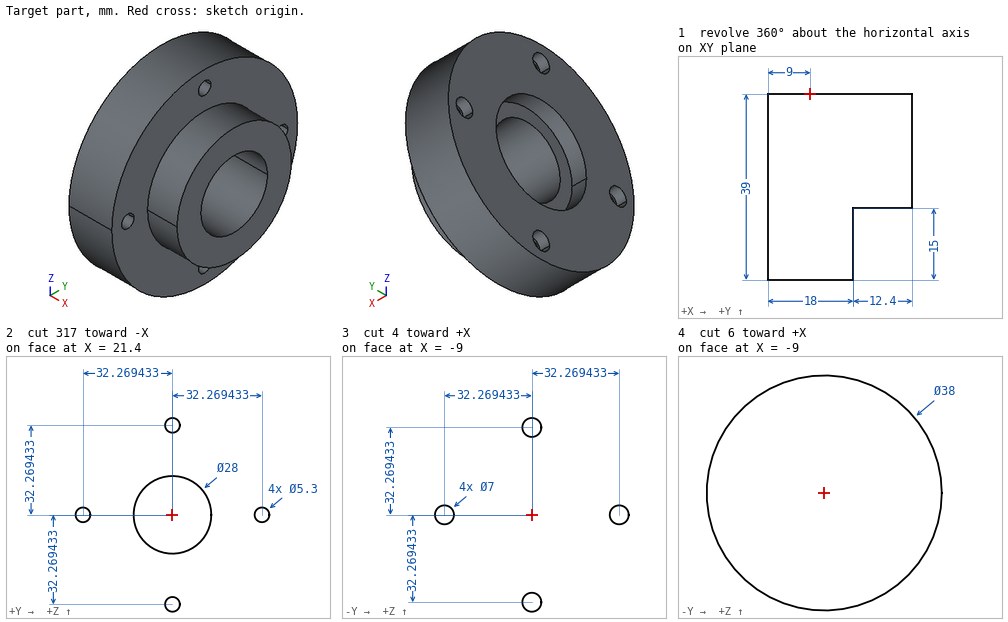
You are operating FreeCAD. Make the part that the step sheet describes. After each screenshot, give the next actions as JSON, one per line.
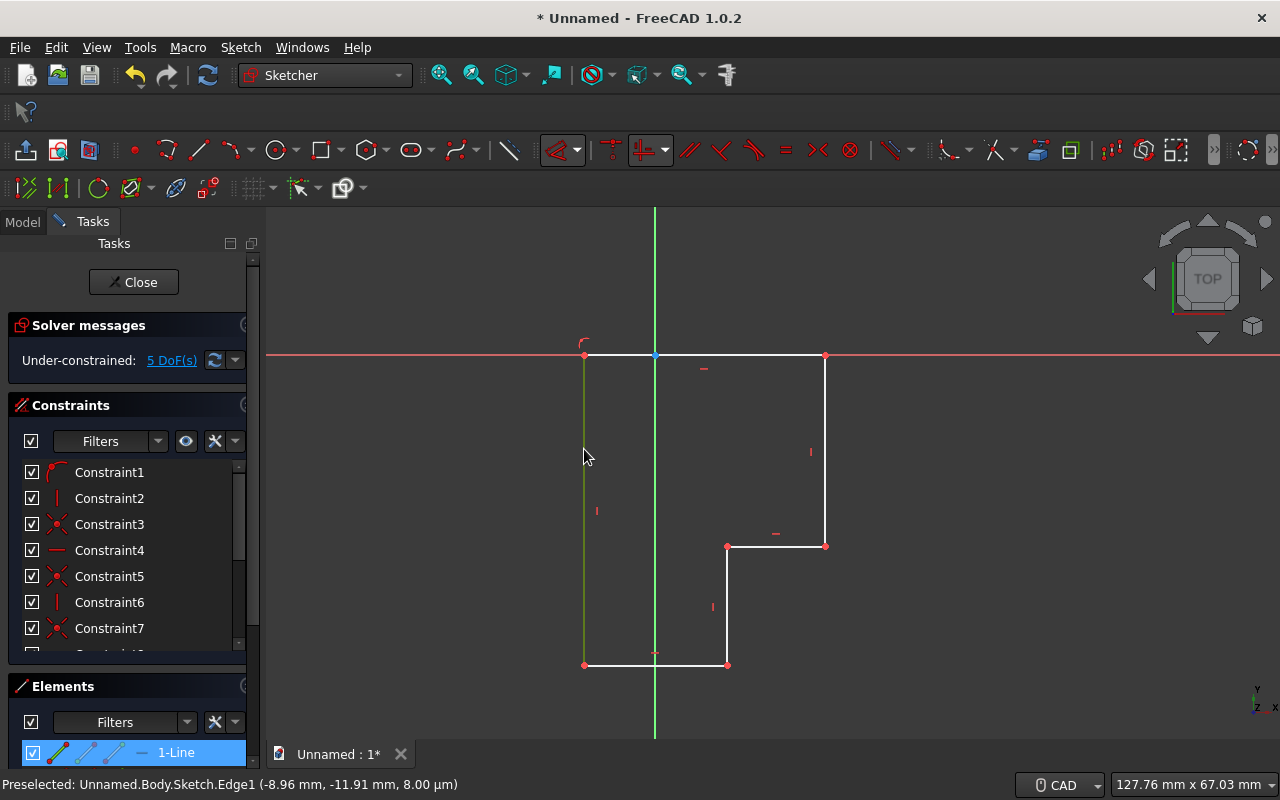
{"action": "left_click", "coordinate": [580, 150]}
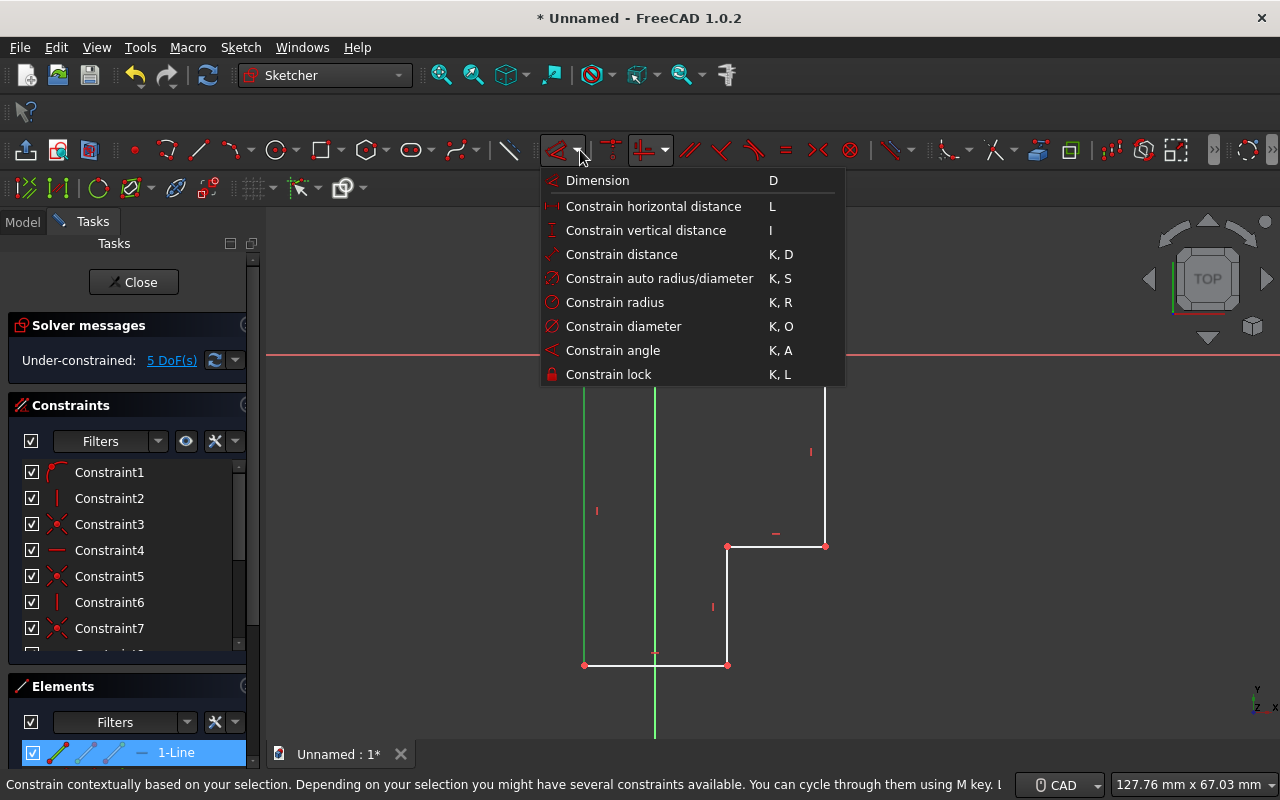
{"action": "left_click", "coordinate": [693, 230]}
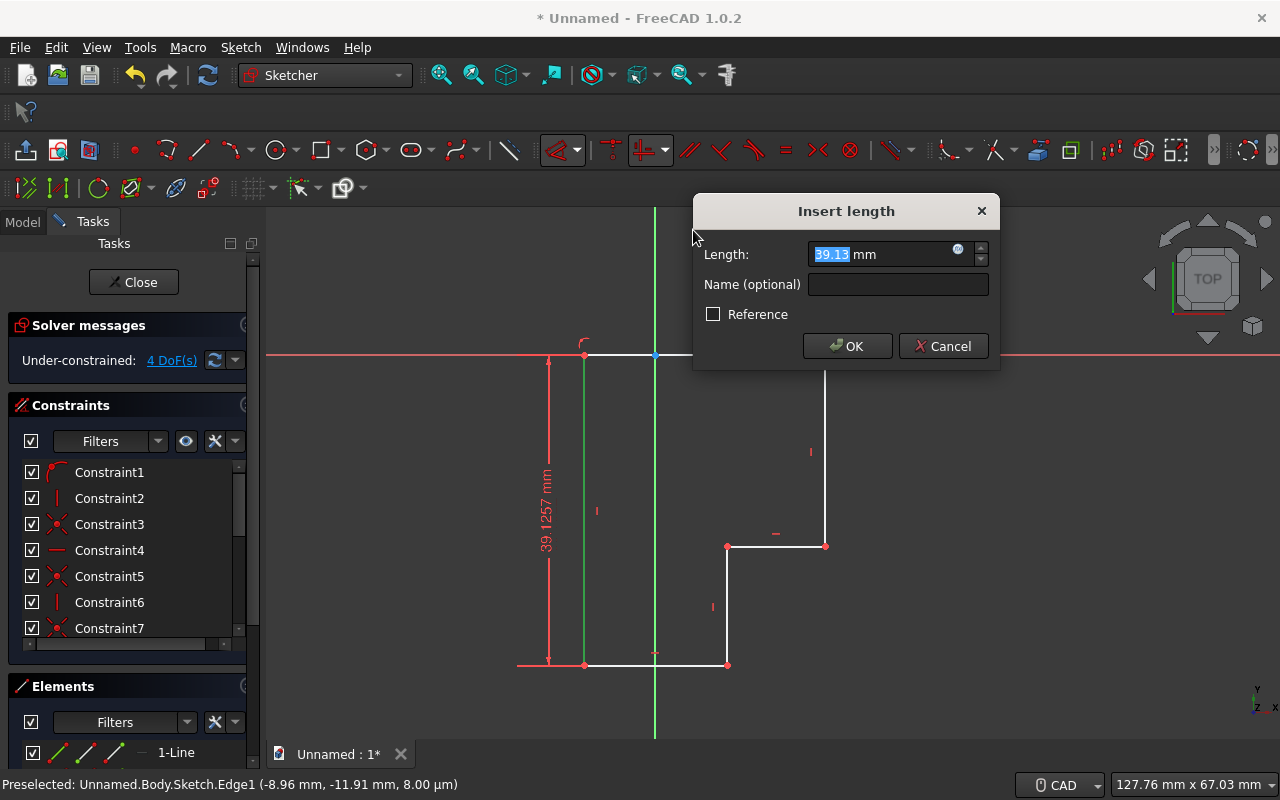
{"action": "type", "text": "39"}
{"action": "key", "text": "Return"}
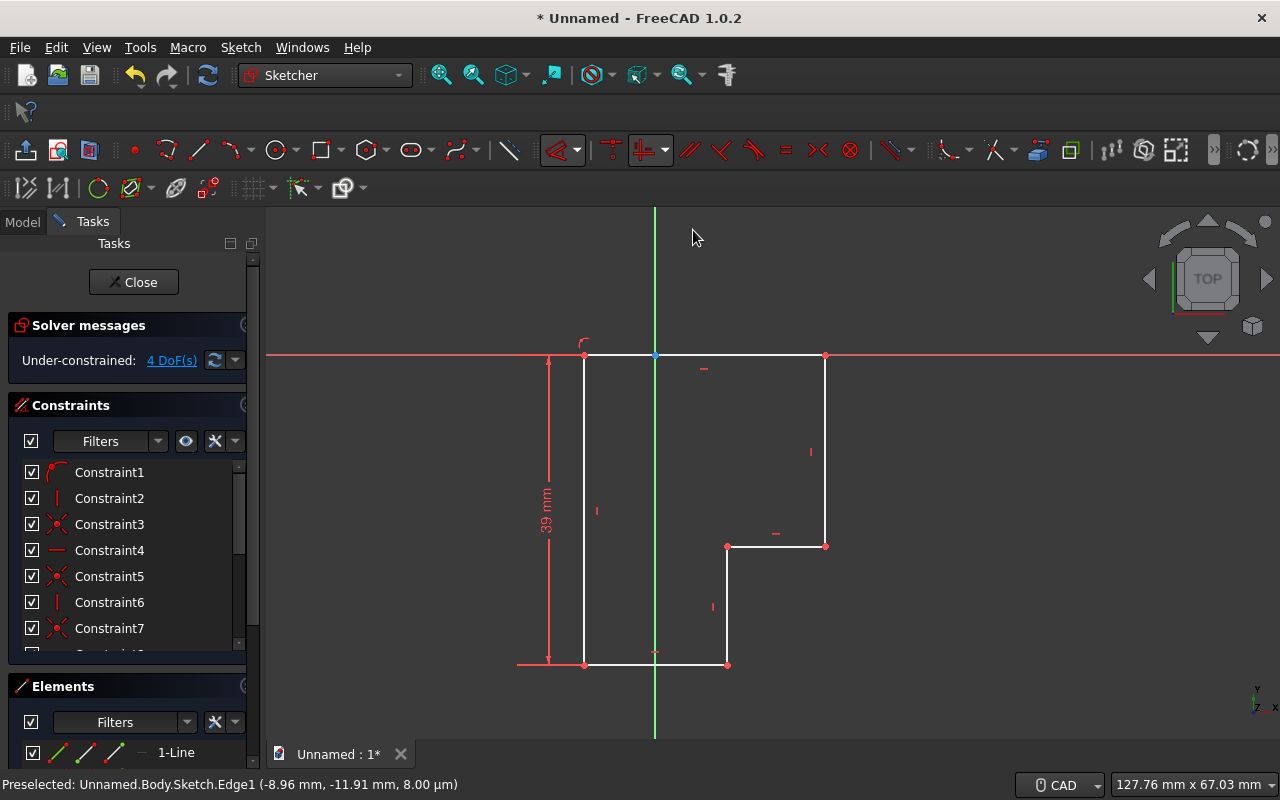
{"action": "left_click", "coordinate": [627, 665]}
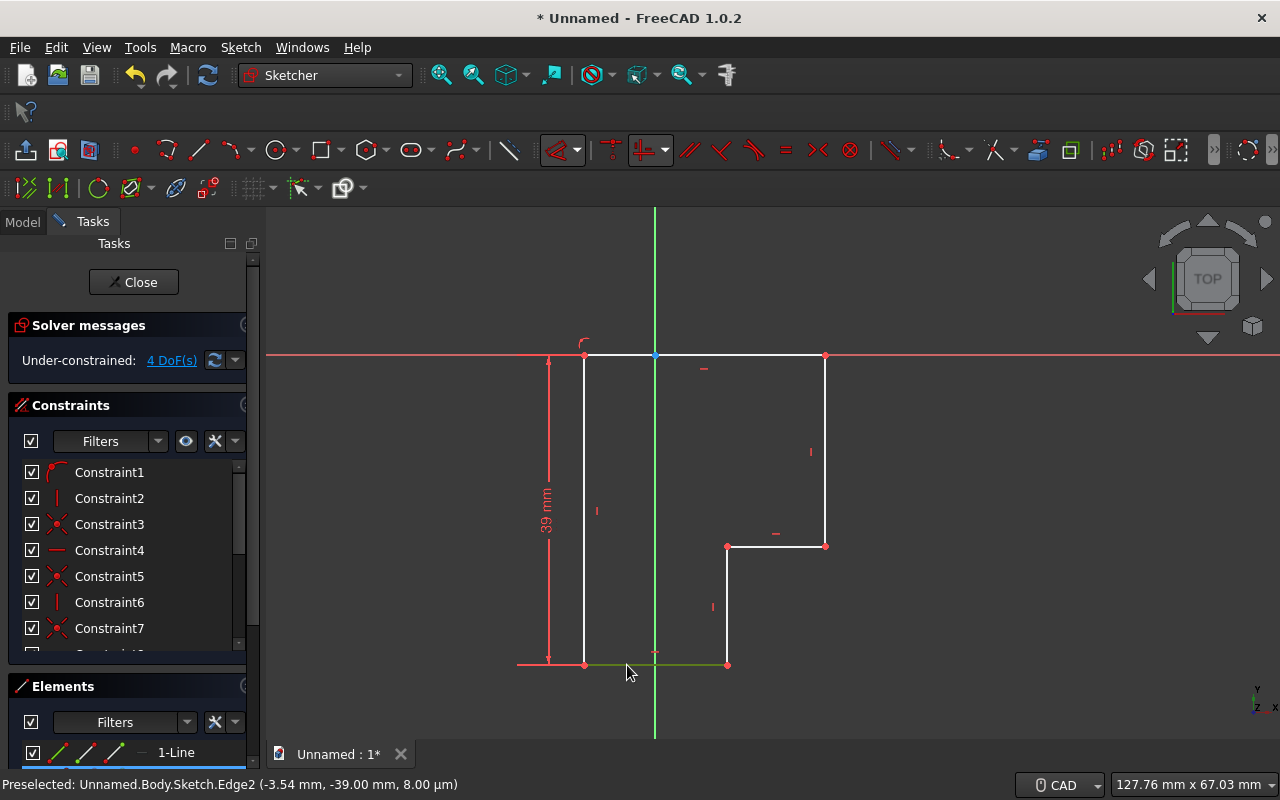
{"action": "key", "text": "l"}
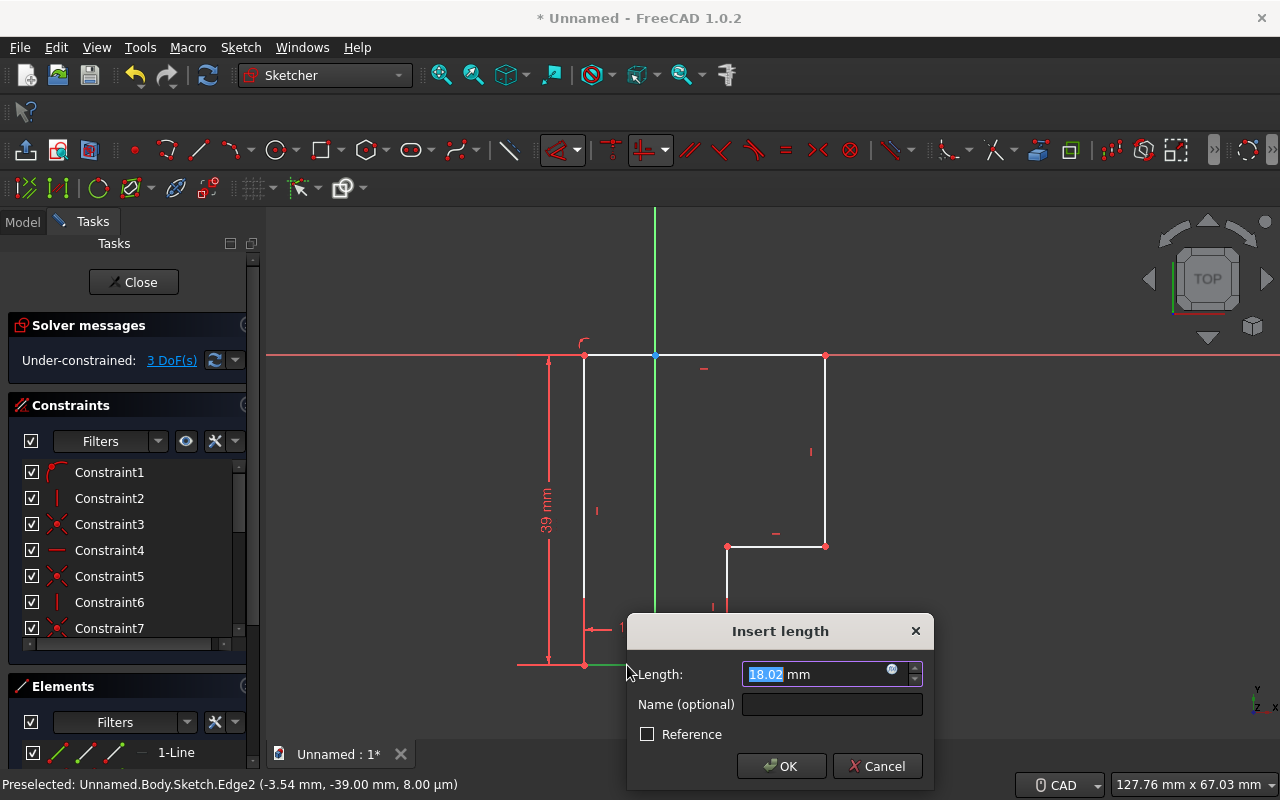
{"action": "type", "text": "18"}
{"action": "key", "text": "Return"}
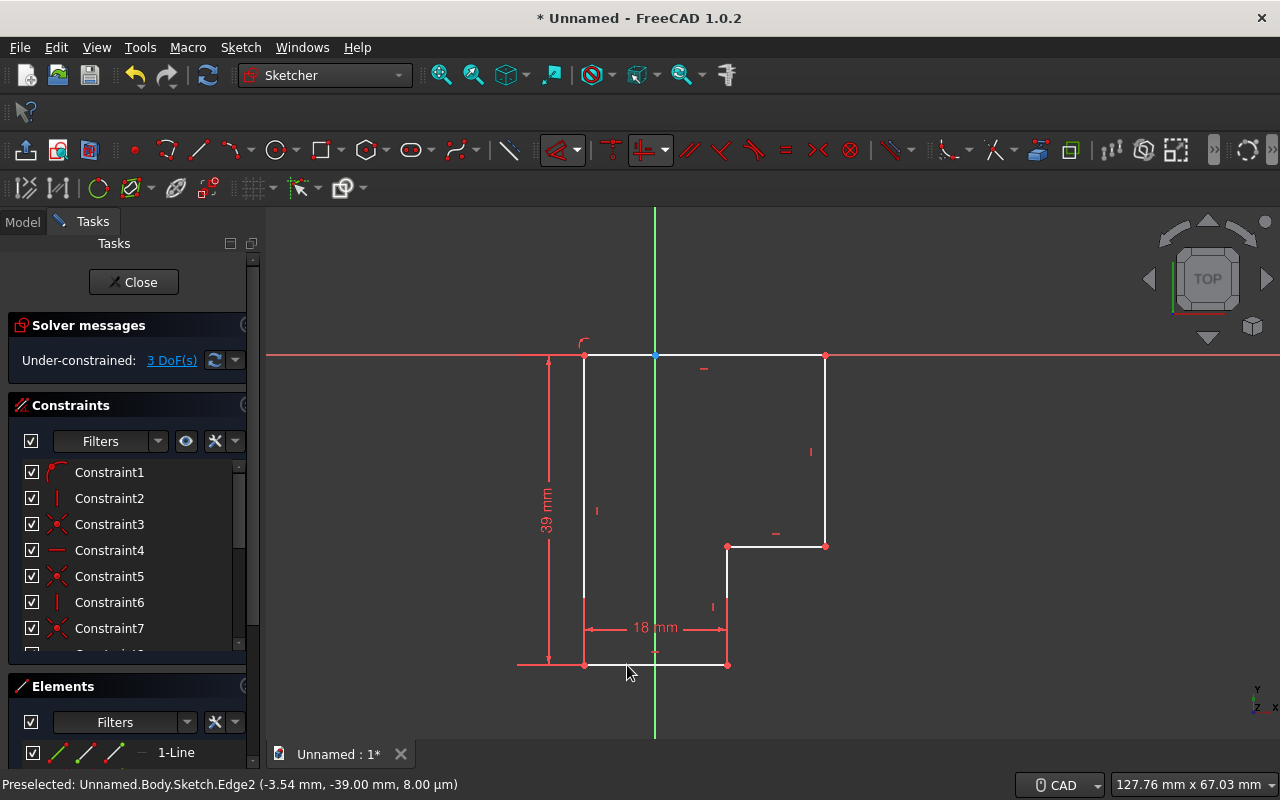
{"action": "left_click", "coordinate": [727, 630]}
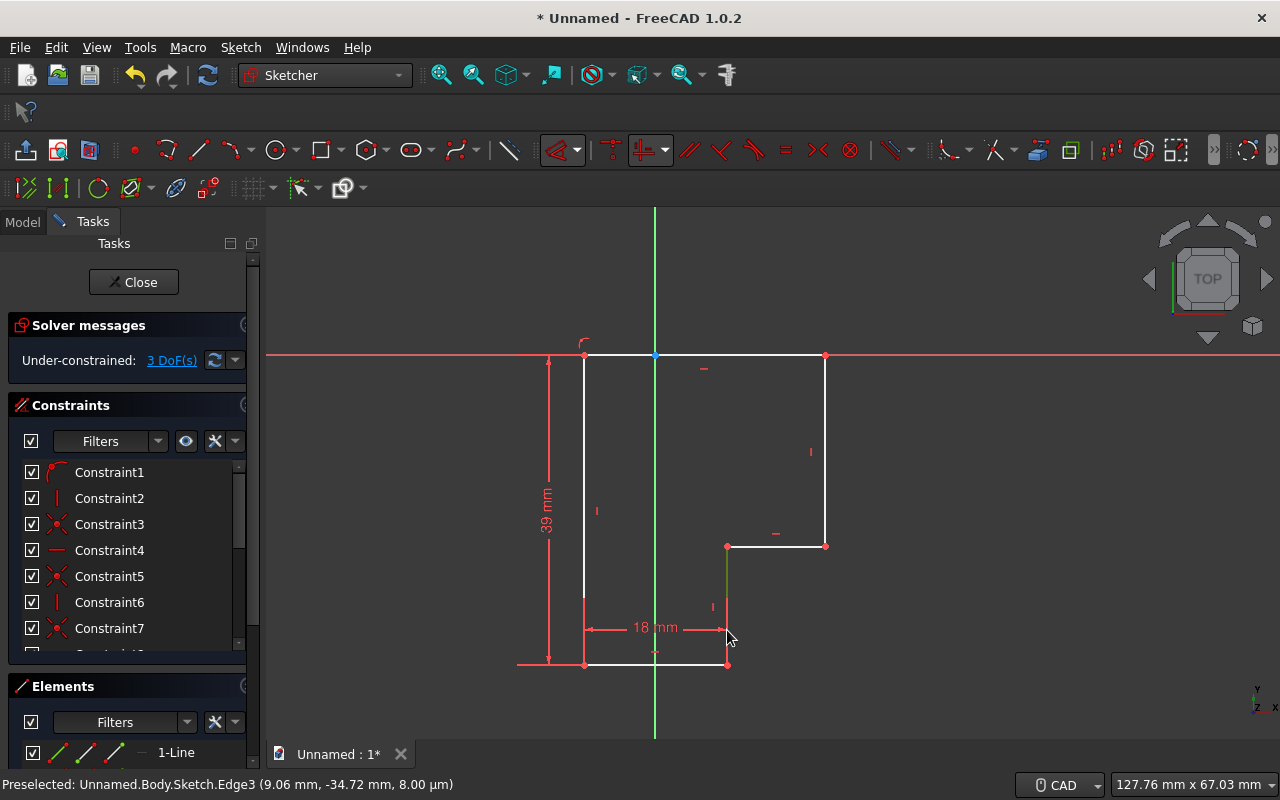
{"action": "left_click", "coordinate": [580, 150]}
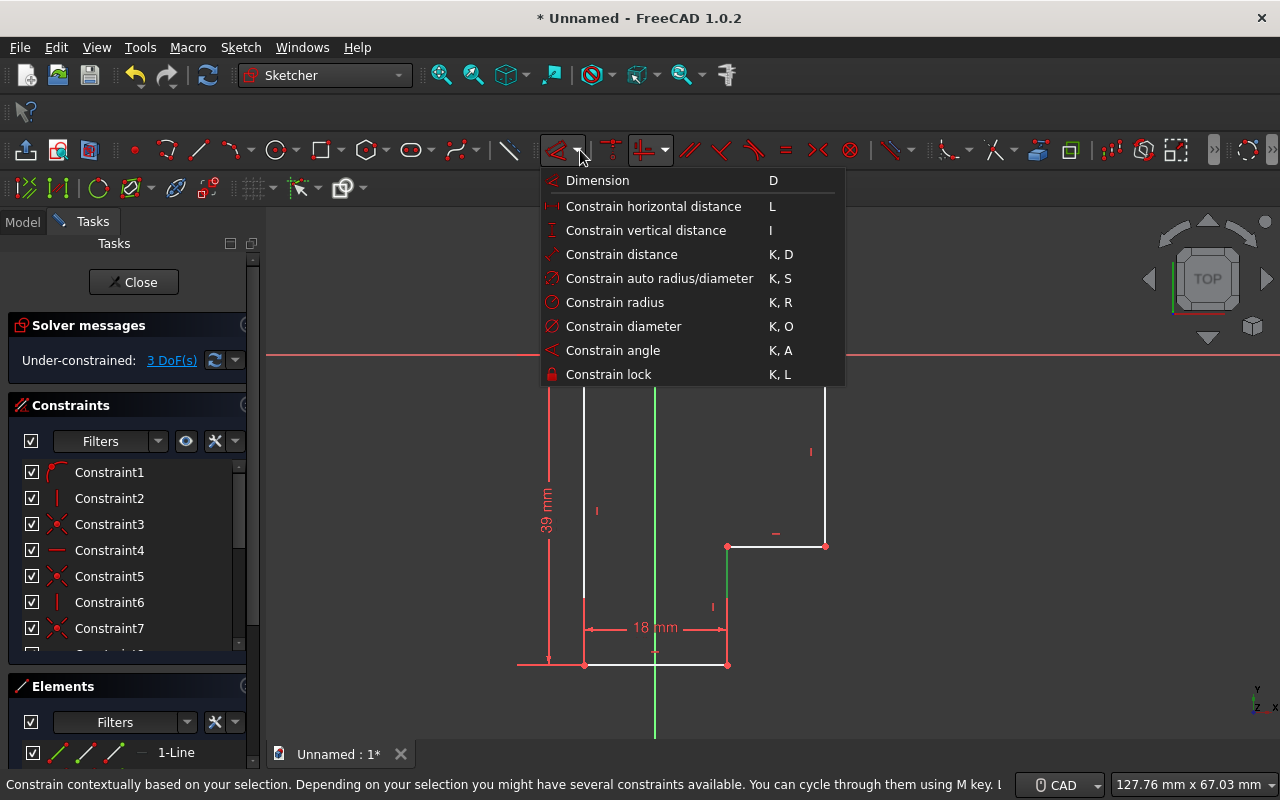
{"action": "left_click", "coordinate": [693, 230]}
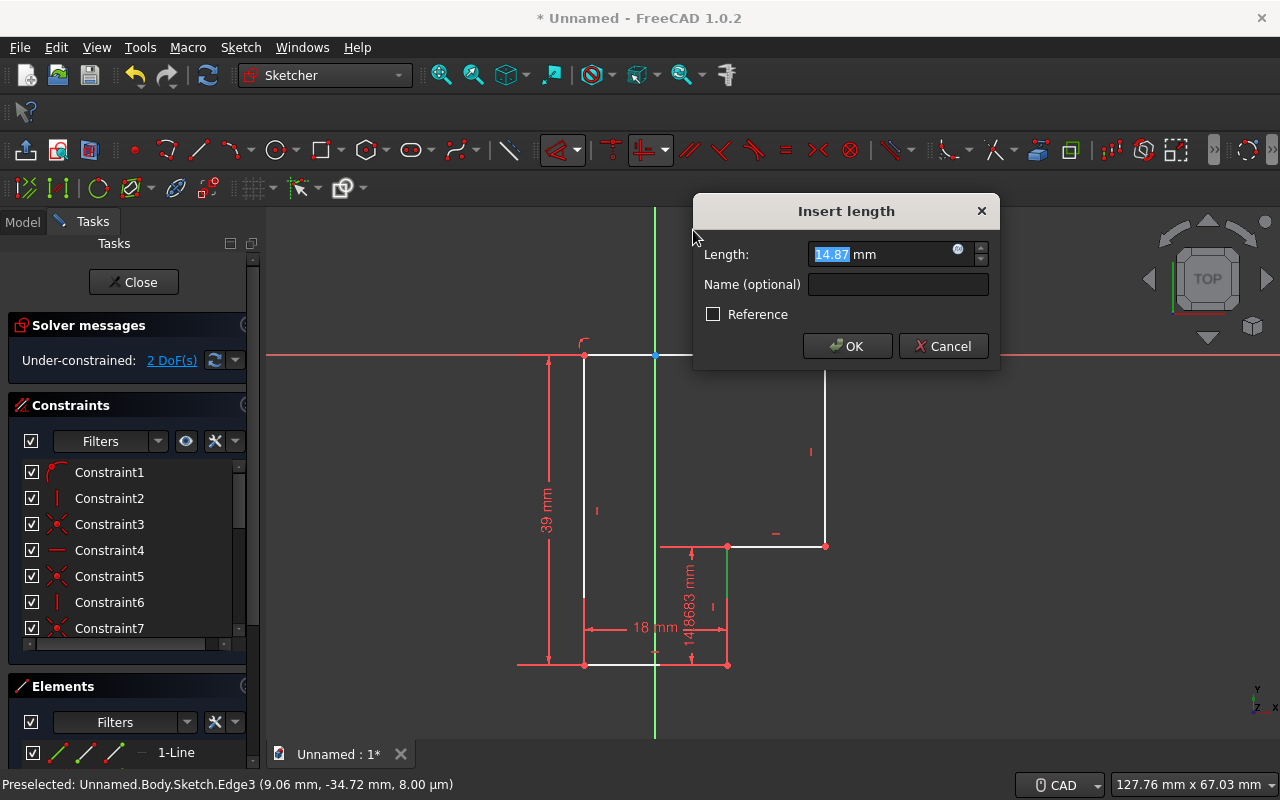
{"action": "type", "text": "15"}
{"action": "key", "text": "Return"}